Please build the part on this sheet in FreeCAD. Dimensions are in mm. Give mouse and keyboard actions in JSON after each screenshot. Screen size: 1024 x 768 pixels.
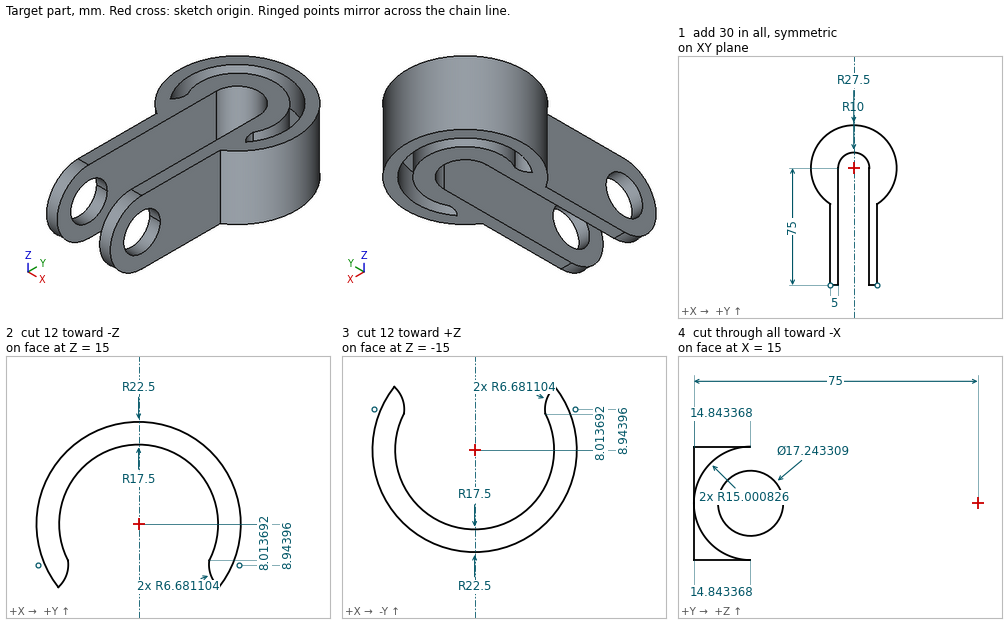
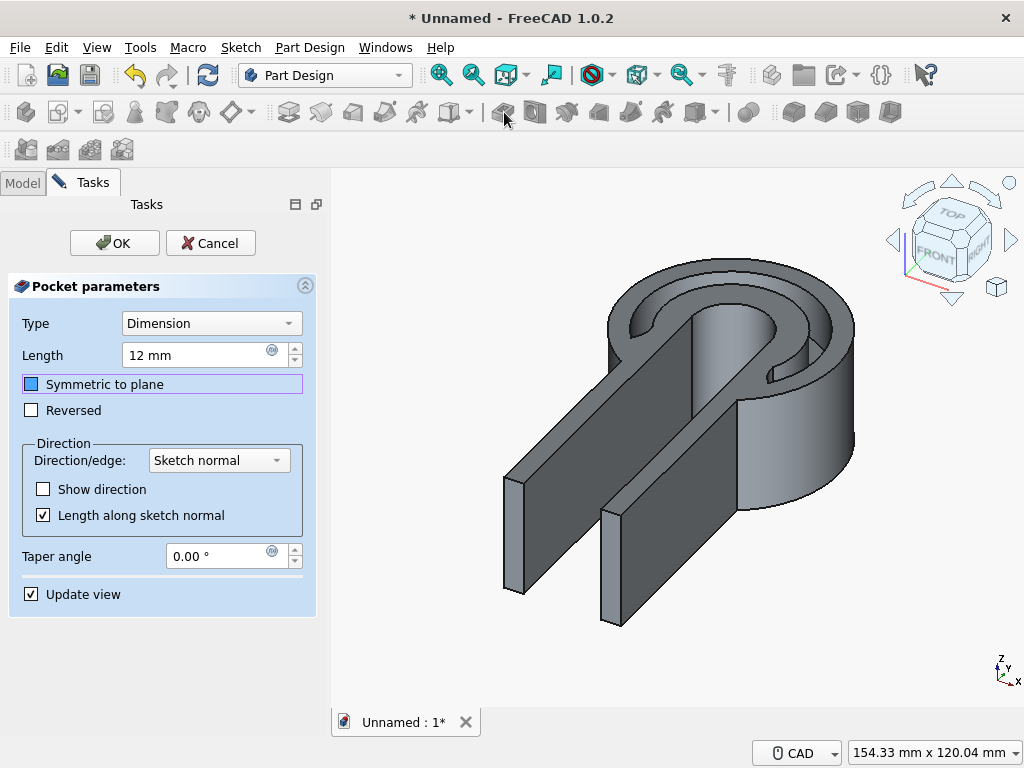
{"action": "left_click", "coordinate": [115, 243]}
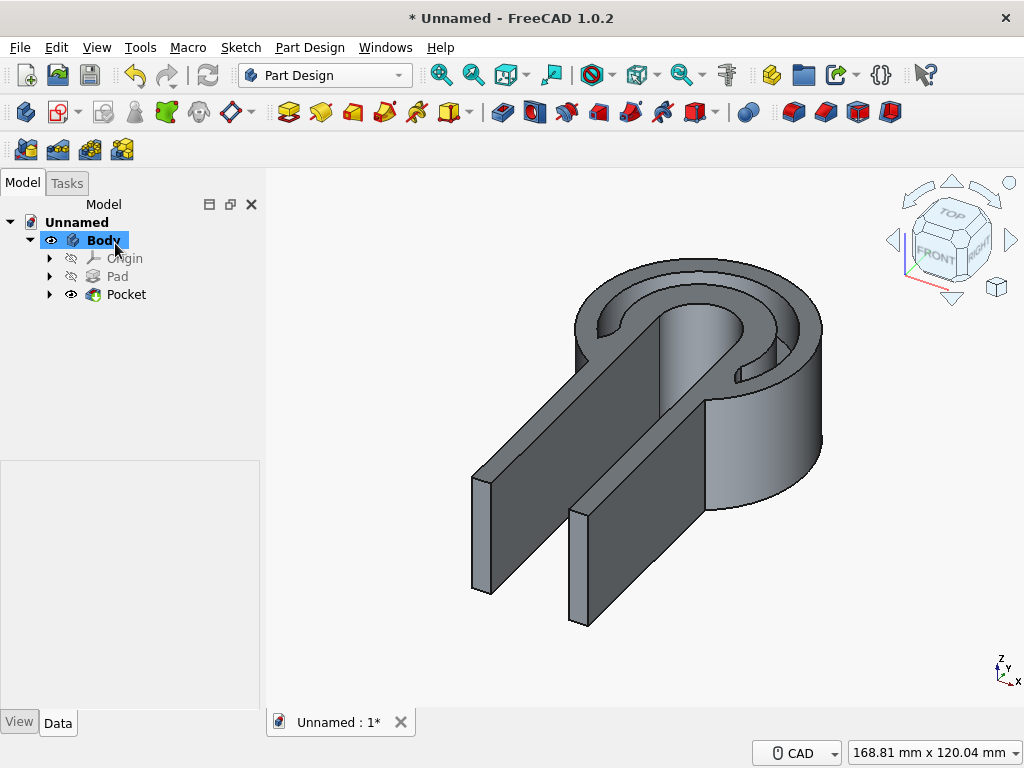
{"action": "key", "text": "5"}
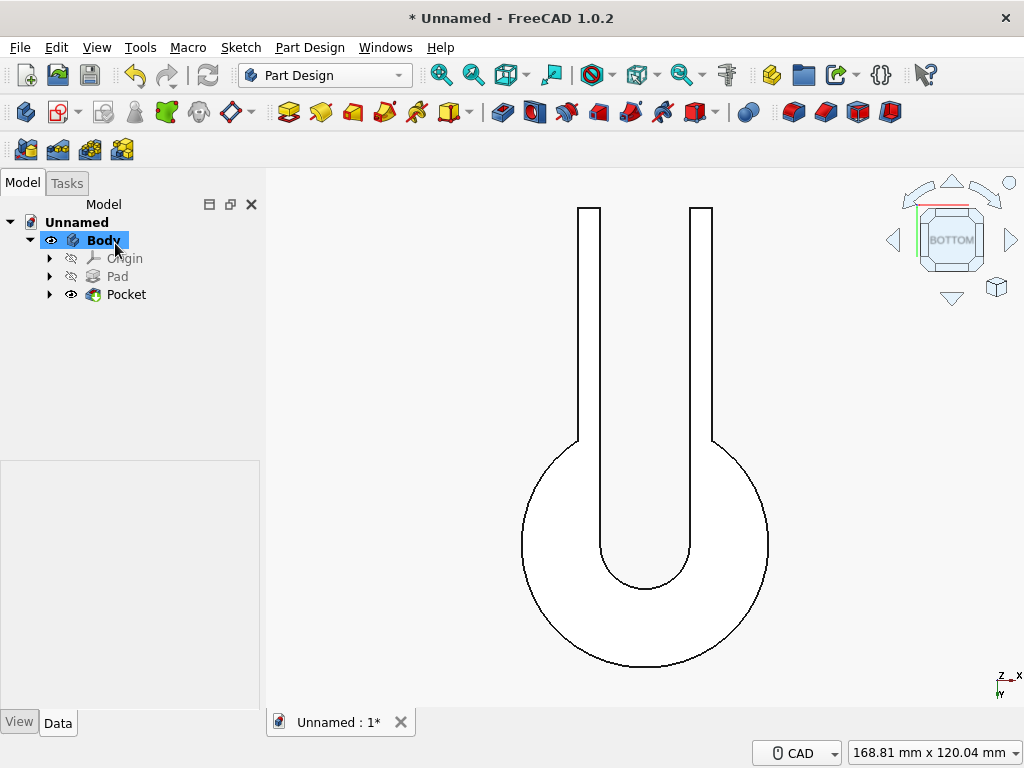
{"action": "left_click", "coordinate": [645, 634]}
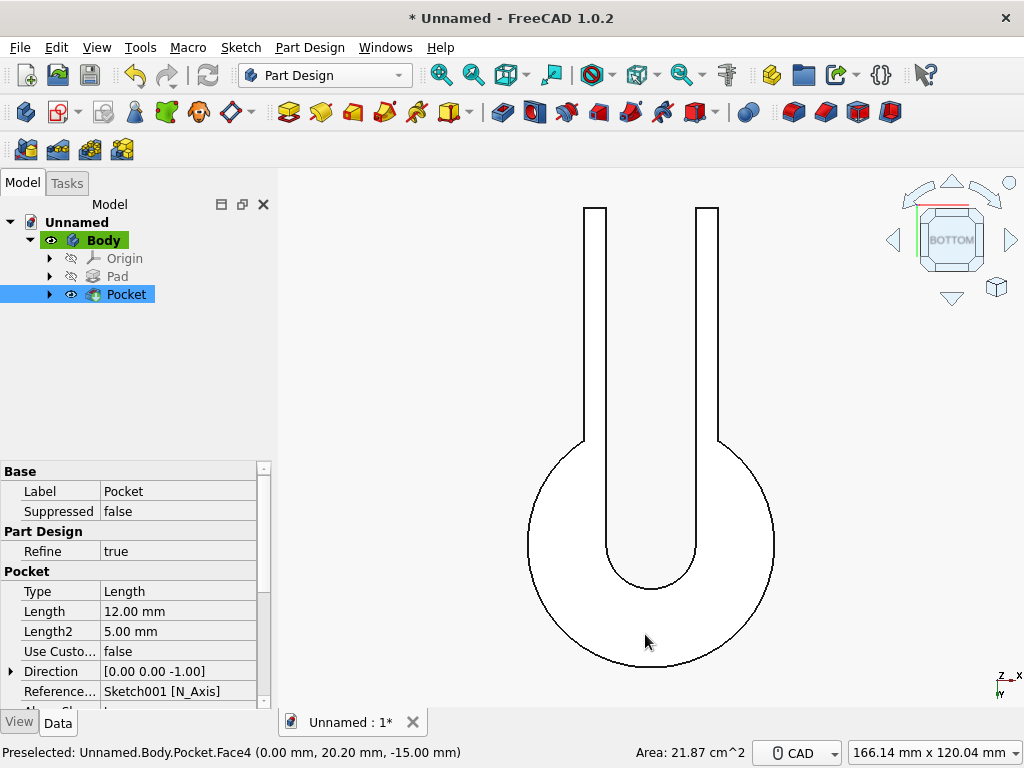
{"action": "left_click", "coordinate": [58, 112]}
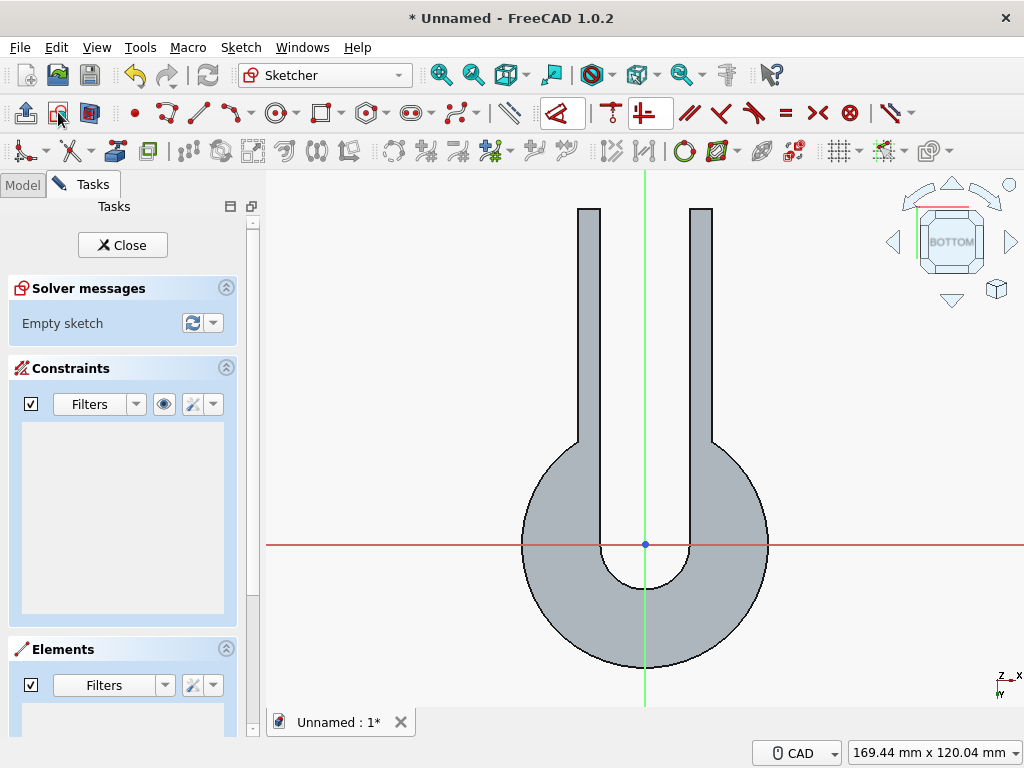
{"action": "scroll", "coordinate": [701, 667], "scroll_direction": "up", "scroll_amount": 4}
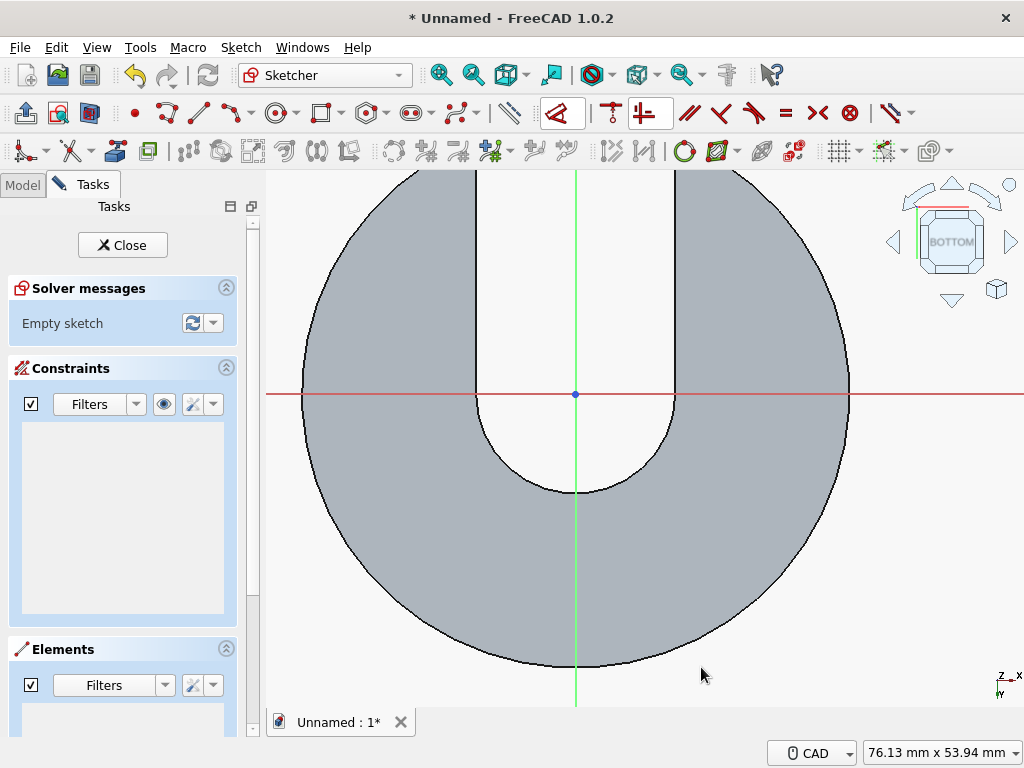
{"action": "key", "text": "g 3 a"}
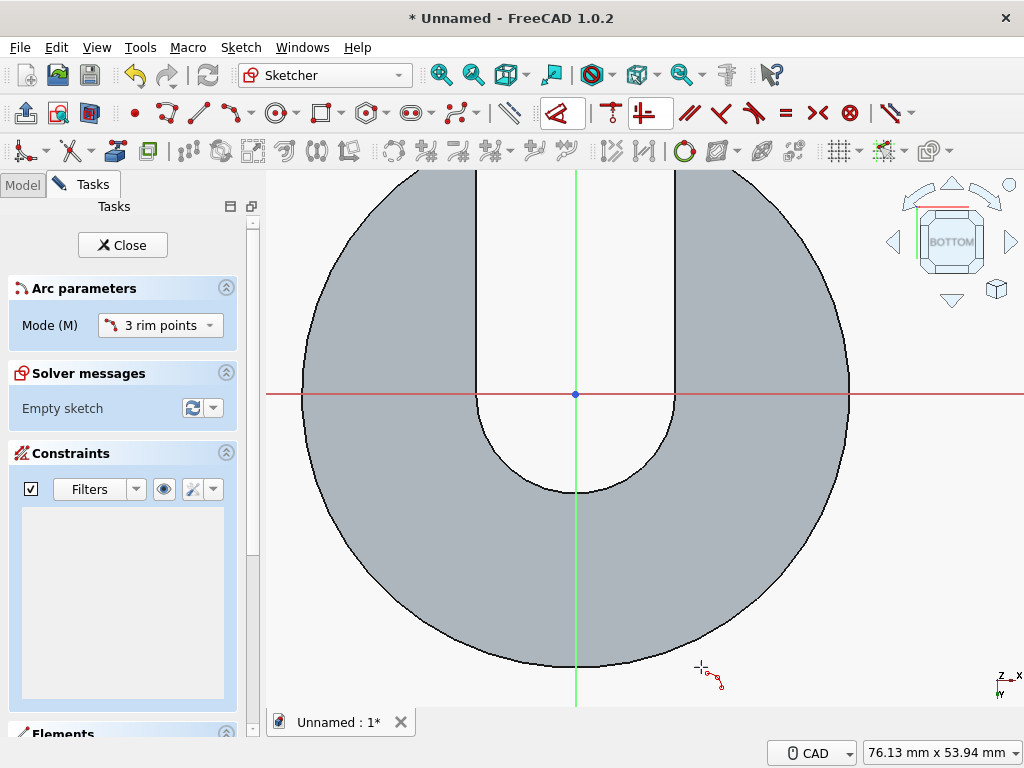
{"action": "left_click", "coordinate": [731, 314]}
{"action": "left_click", "coordinate": [752, 256]}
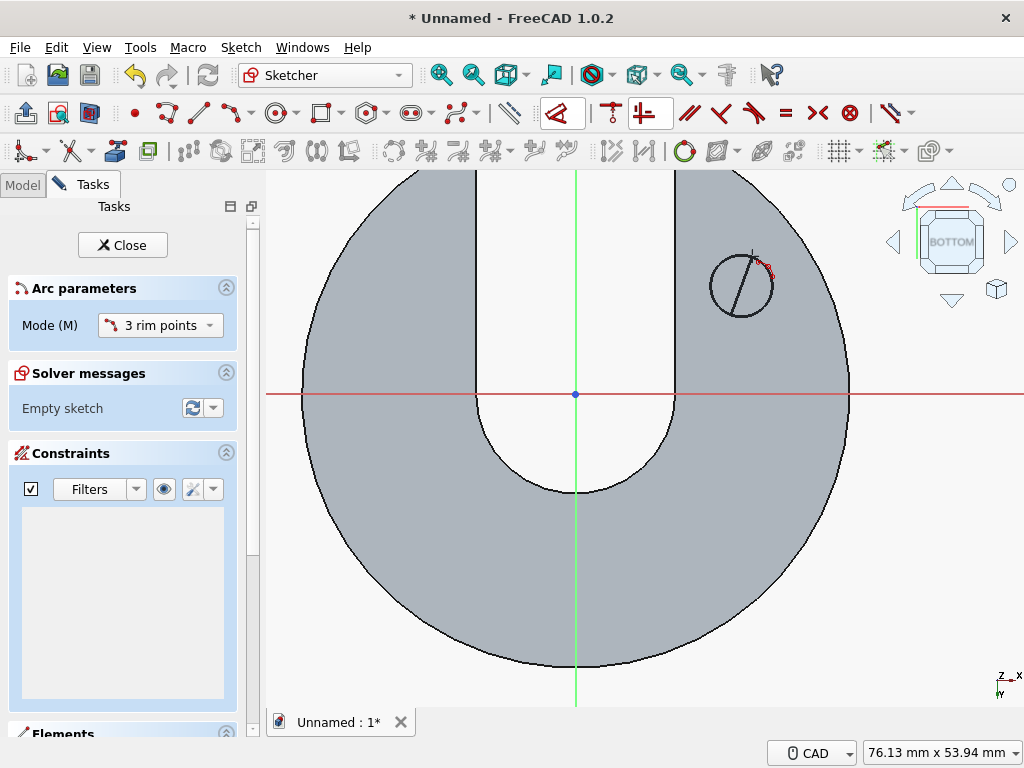
{"action": "scroll", "coordinate": [734, 282], "scroll_direction": "up", "scroll_amount": 4}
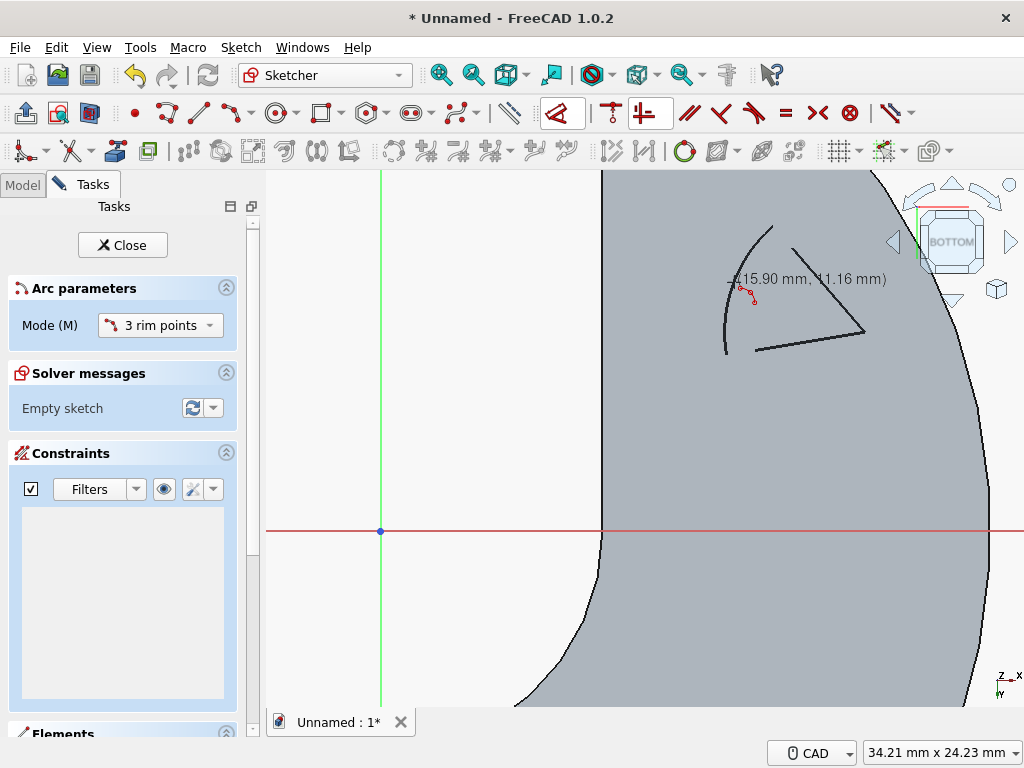
{"action": "left_click", "coordinate": [733, 283]}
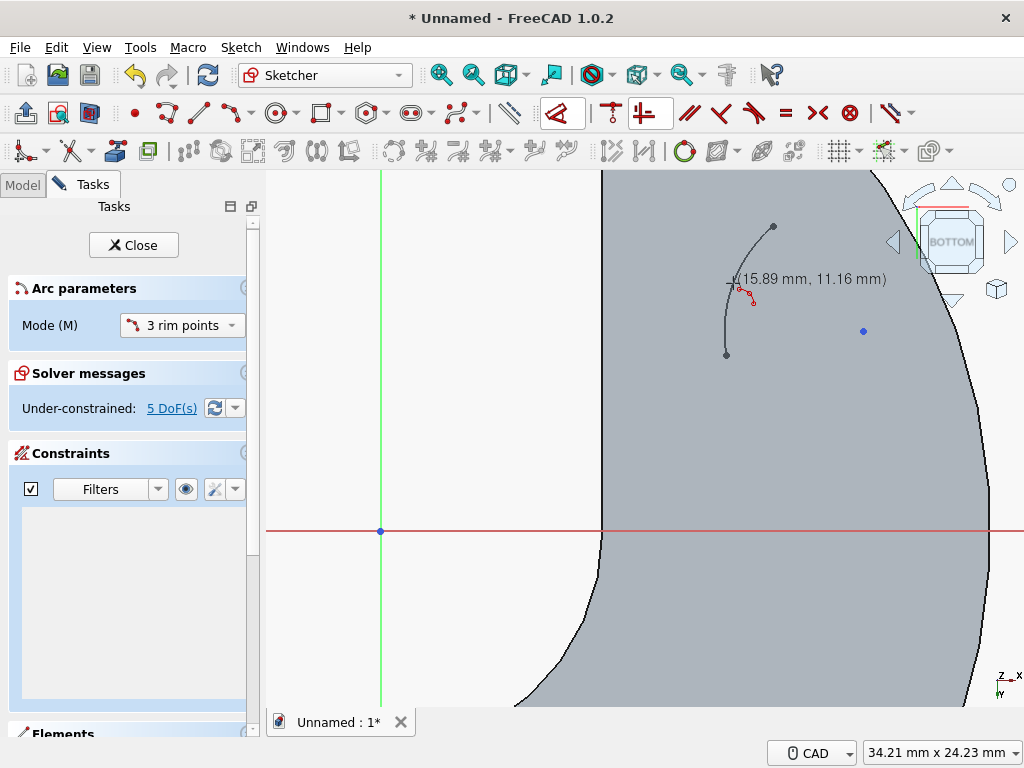
{"action": "left_click", "coordinate": [773, 226]}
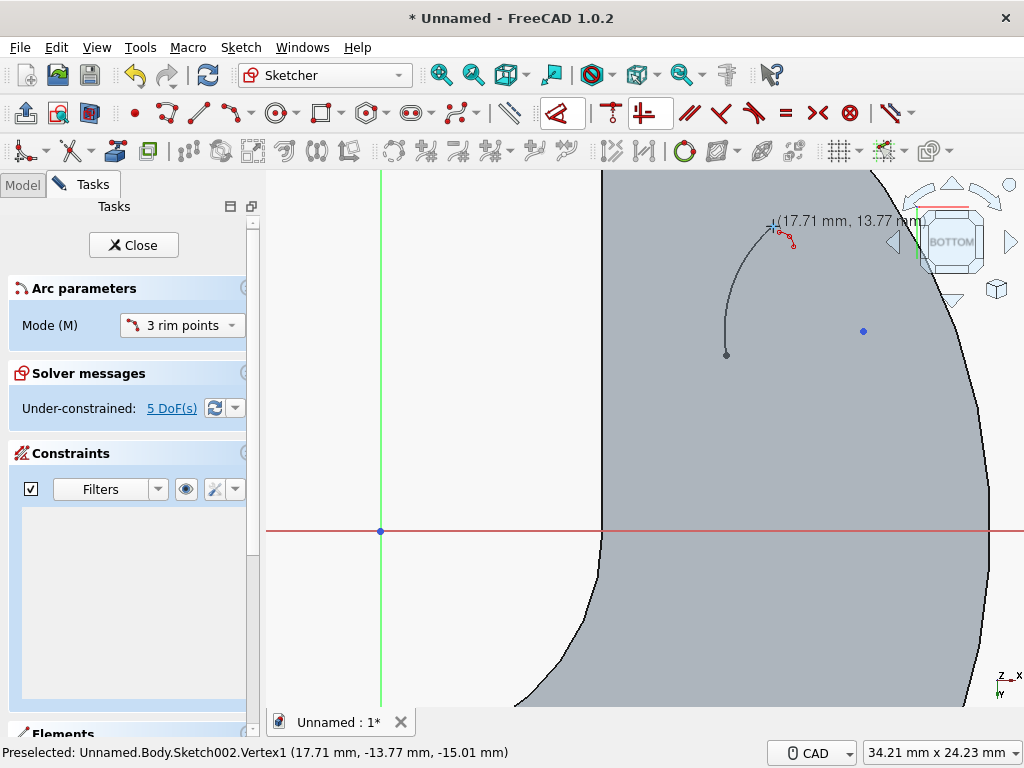
{"action": "scroll", "coordinate": [736, 285], "scroll_direction": "down", "scroll_amount": 4}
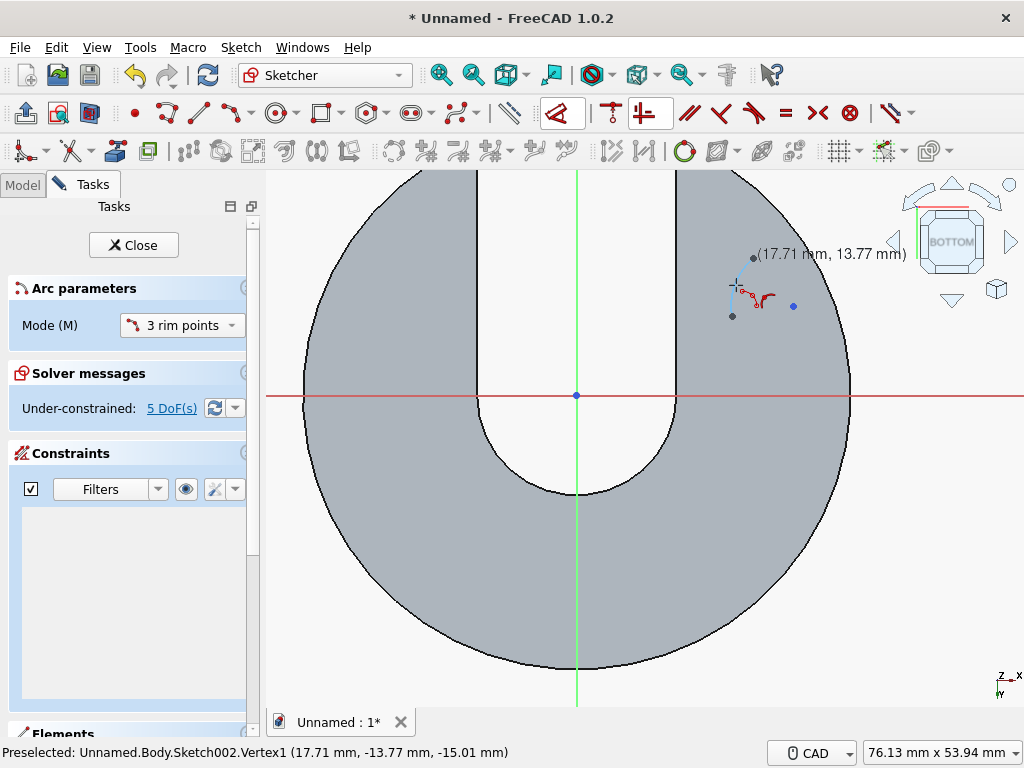
{"action": "left_click", "coordinate": [401, 257]}
{"action": "left_click", "coordinate": [480, 598]}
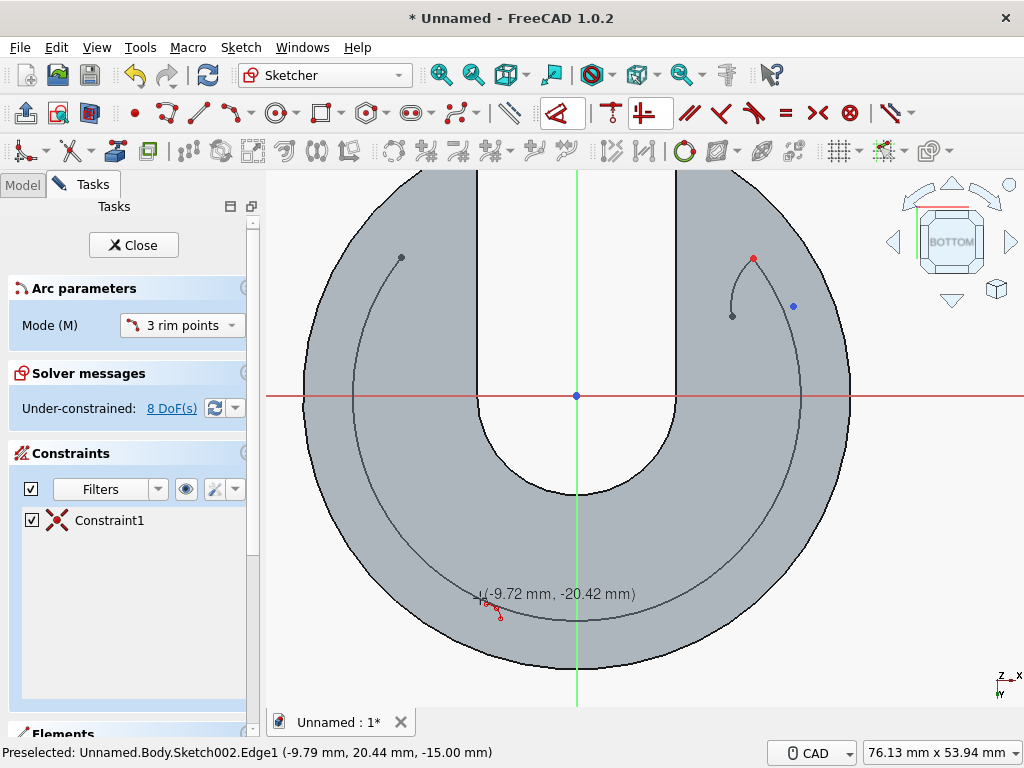
{"action": "left_click", "coordinate": [401, 258]}
{"action": "left_click", "coordinate": [422, 316]}